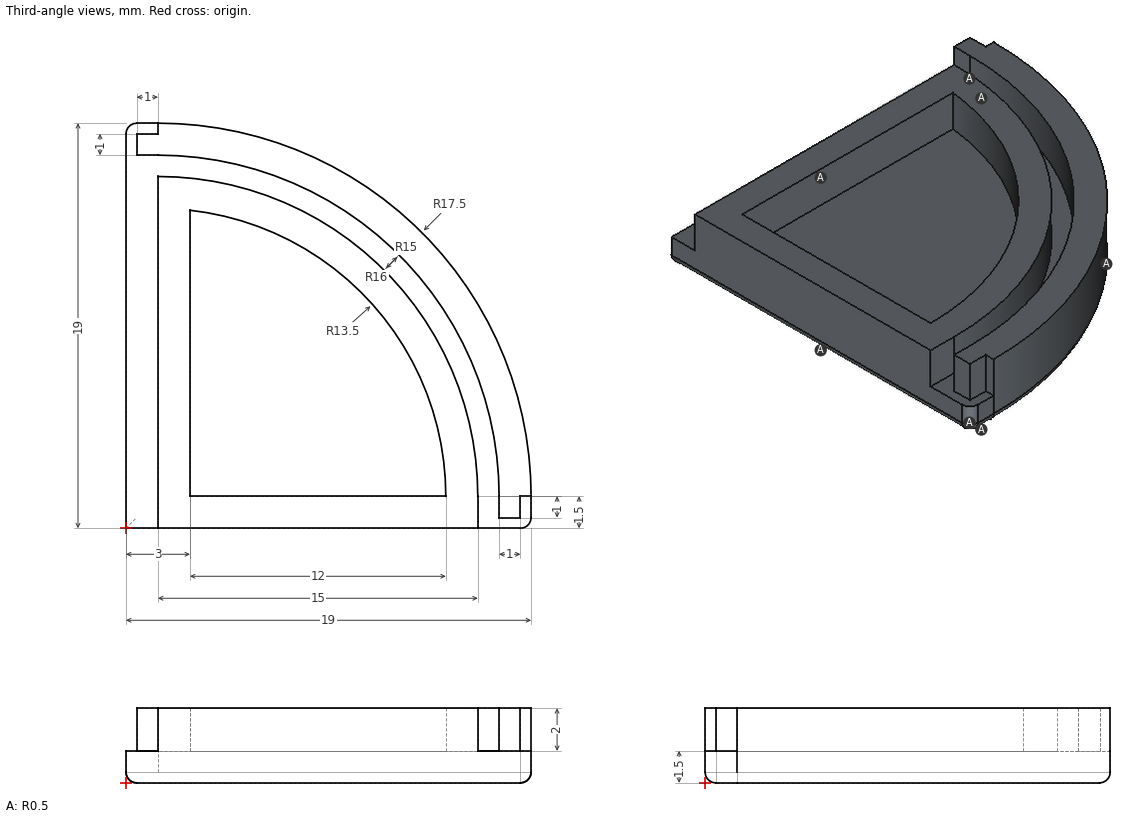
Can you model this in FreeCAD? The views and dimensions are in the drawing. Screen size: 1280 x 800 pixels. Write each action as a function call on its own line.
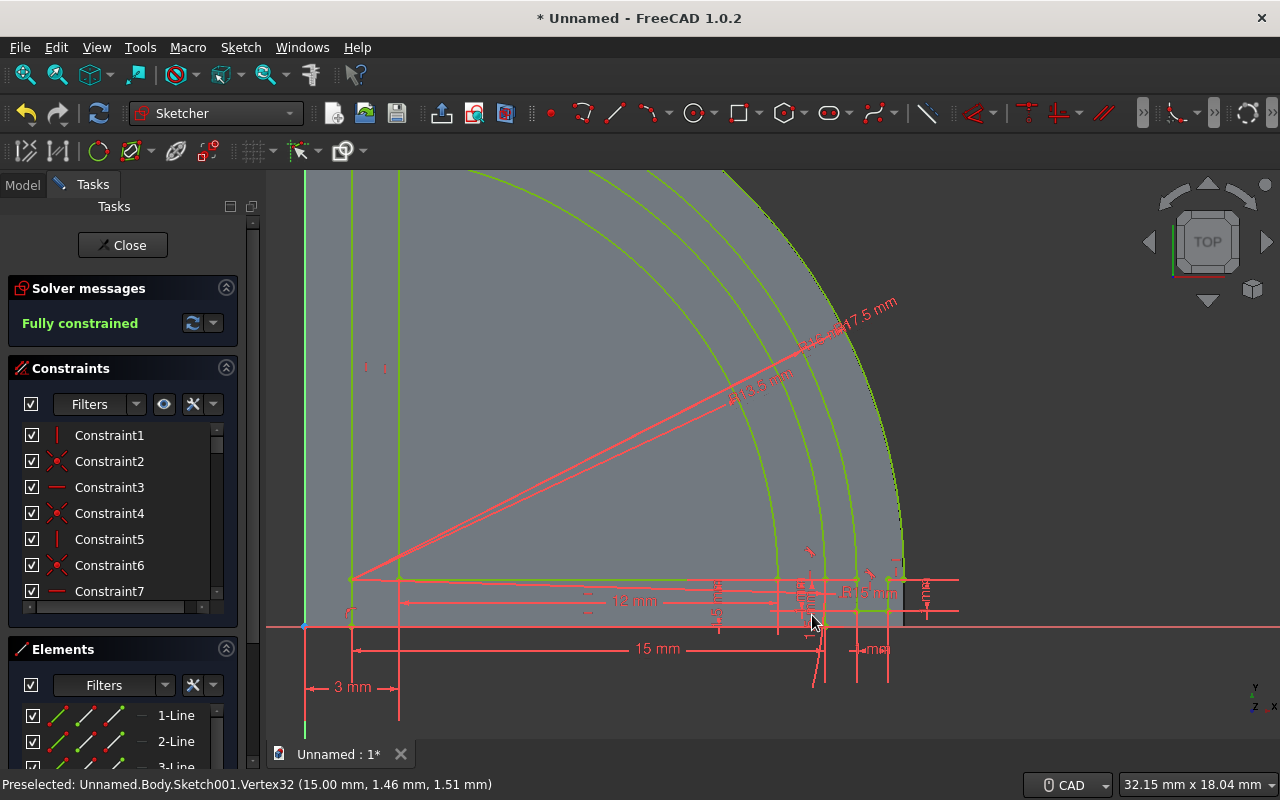
click(123, 245)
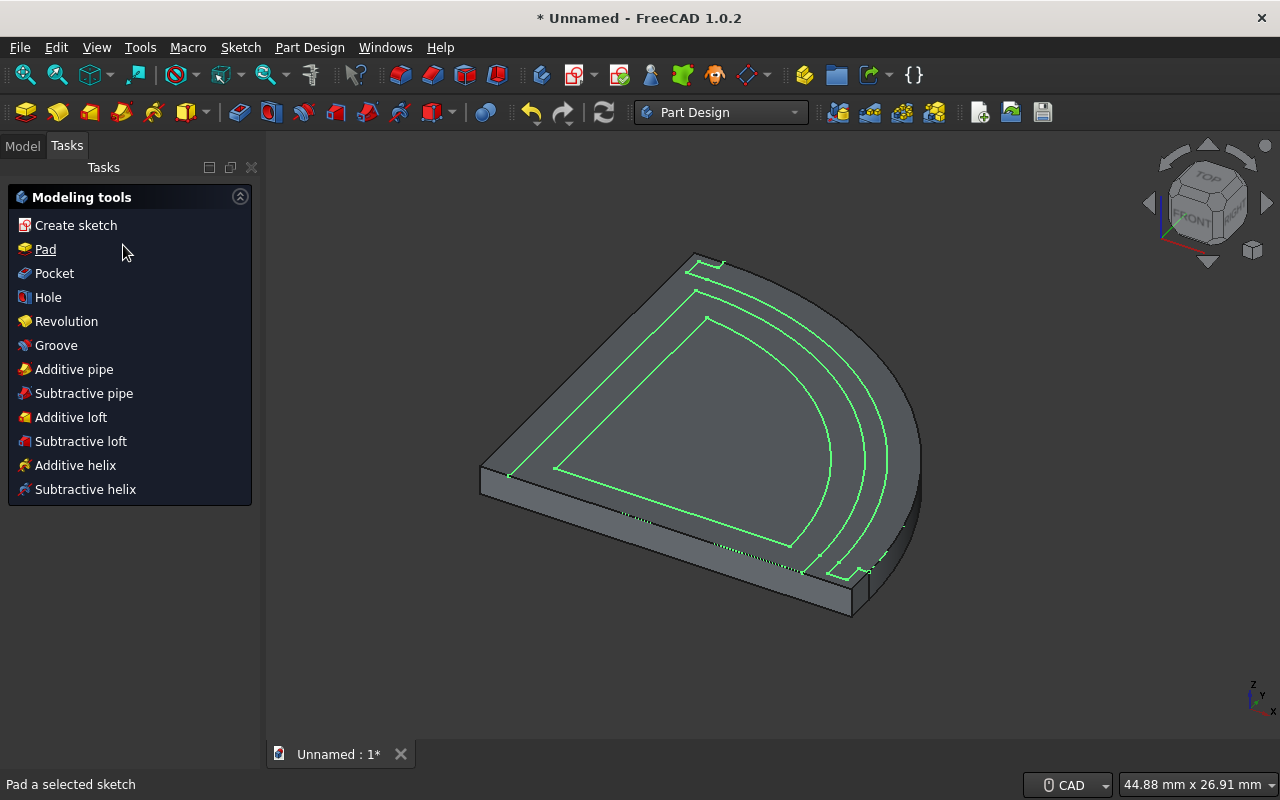
click(26, 112)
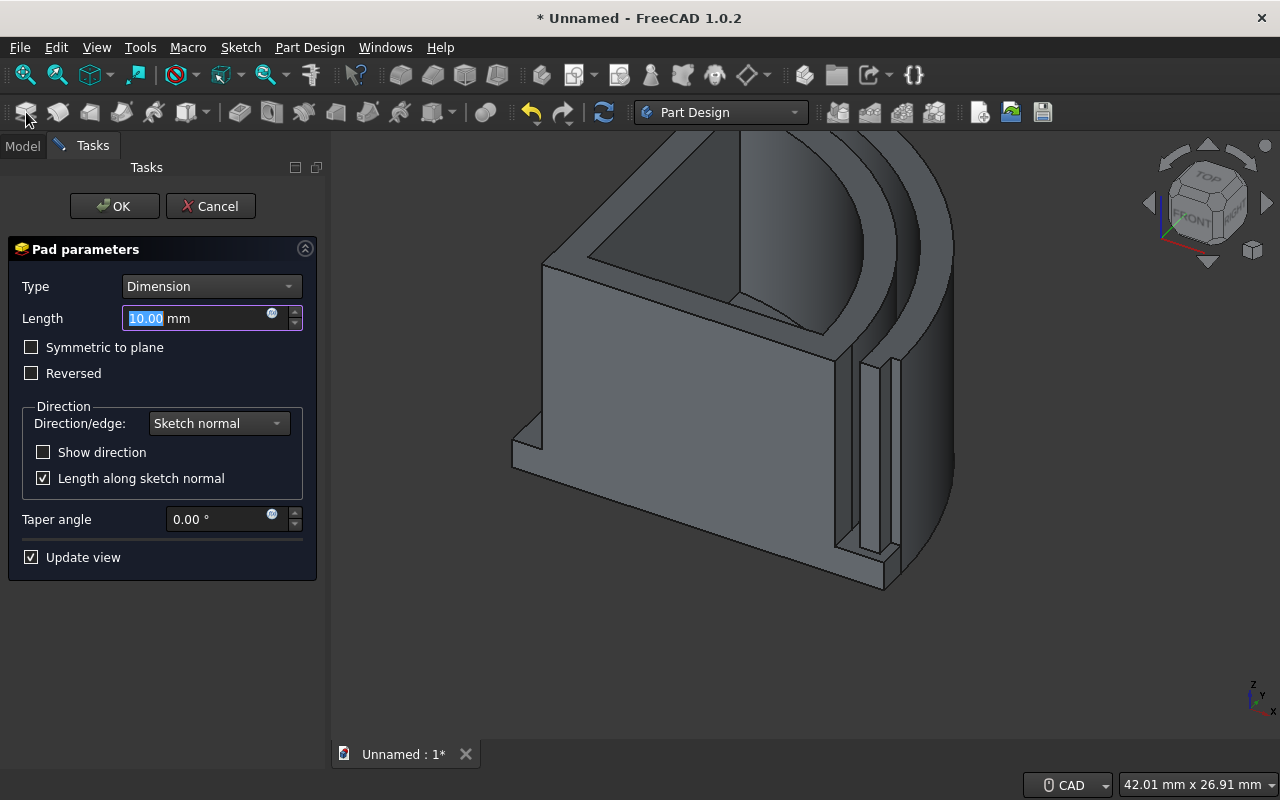
text(2)
key(Tab)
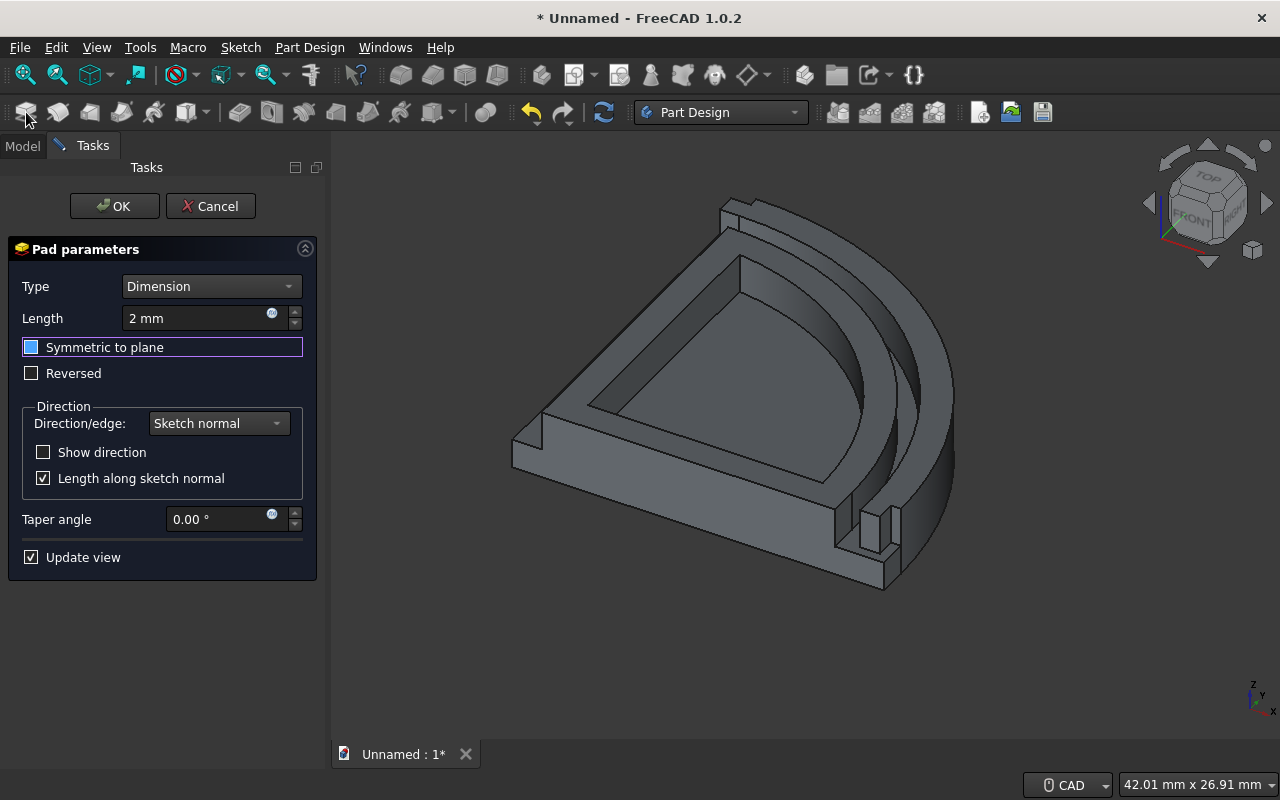
click(115, 206)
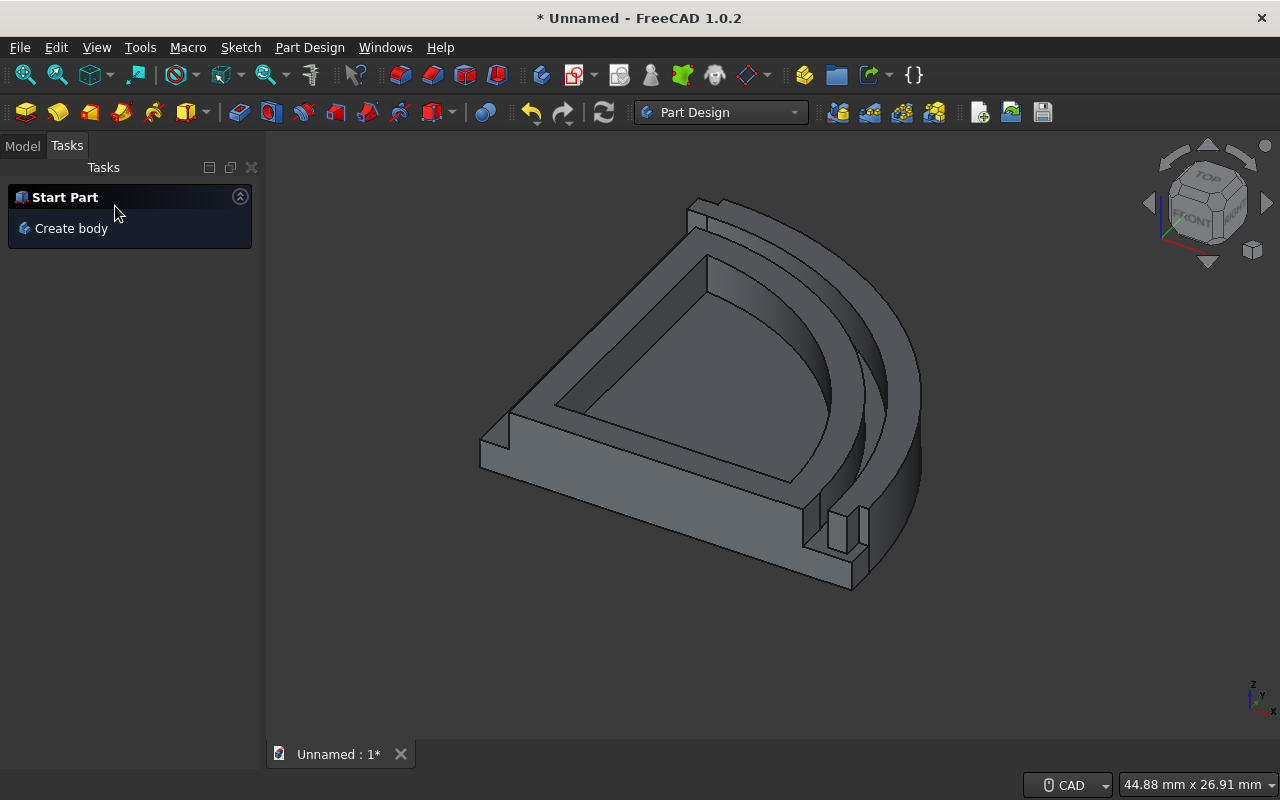
click(852, 576)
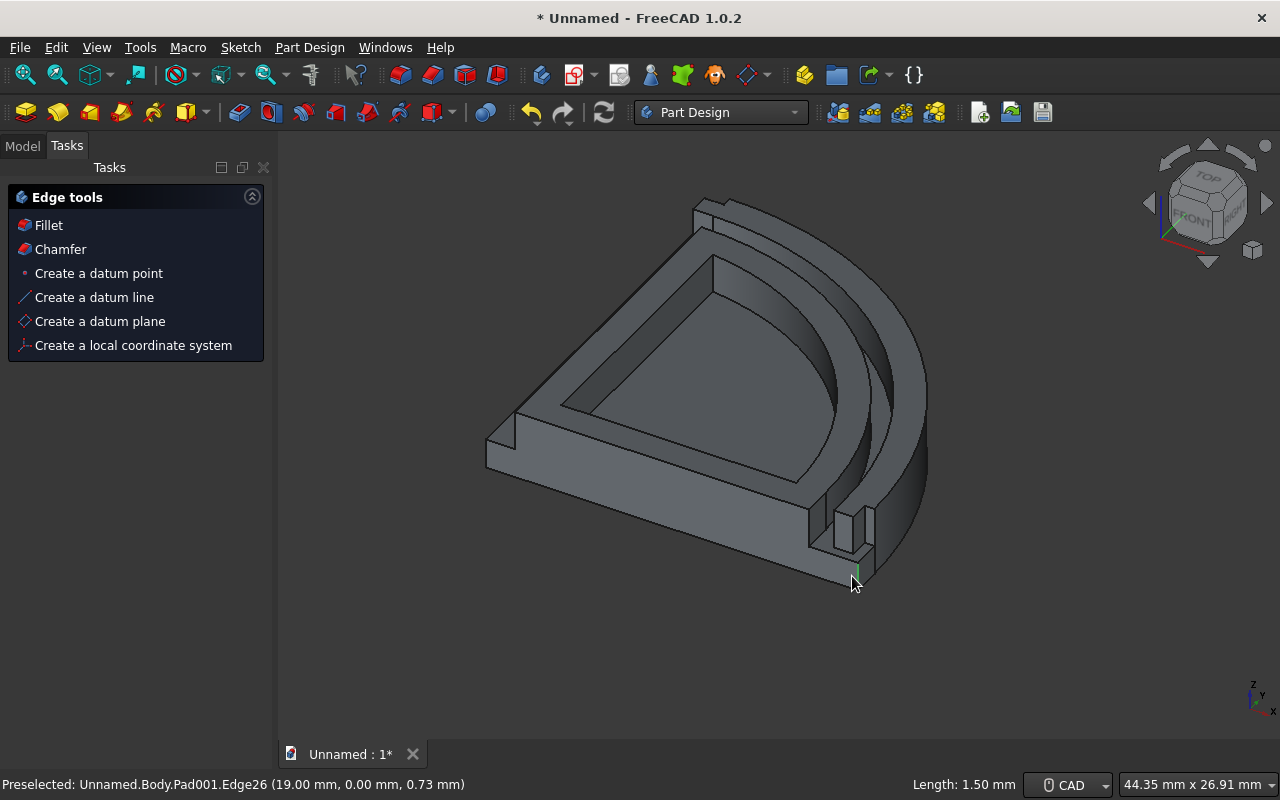
key(0)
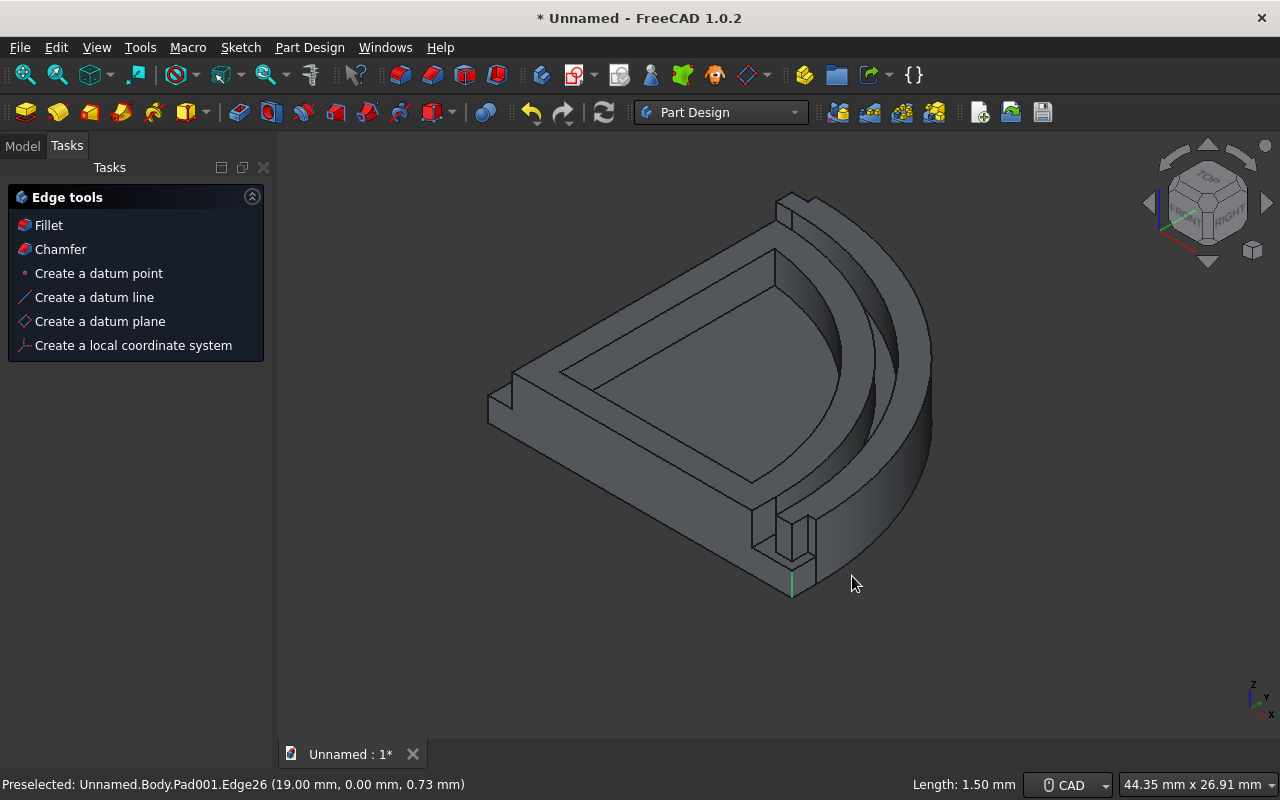
key(2)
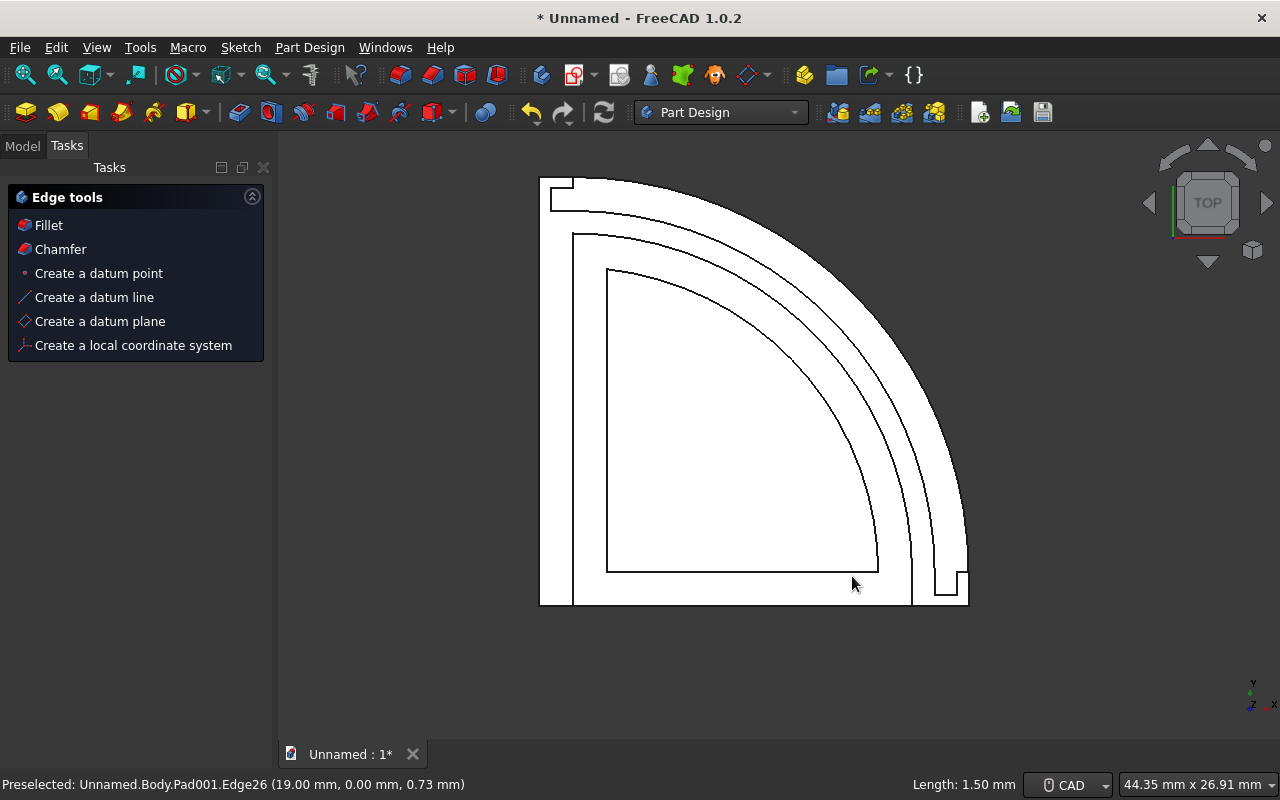
key(1)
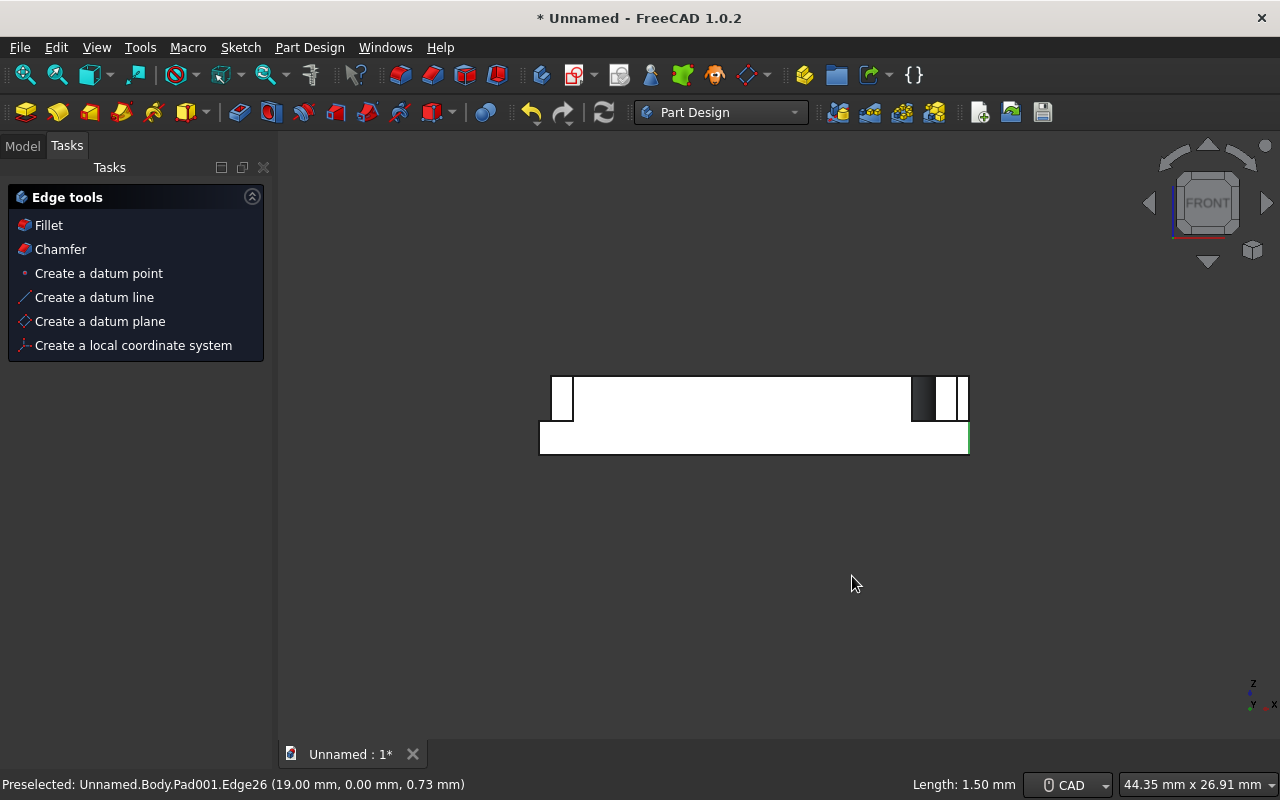
click(26, 76)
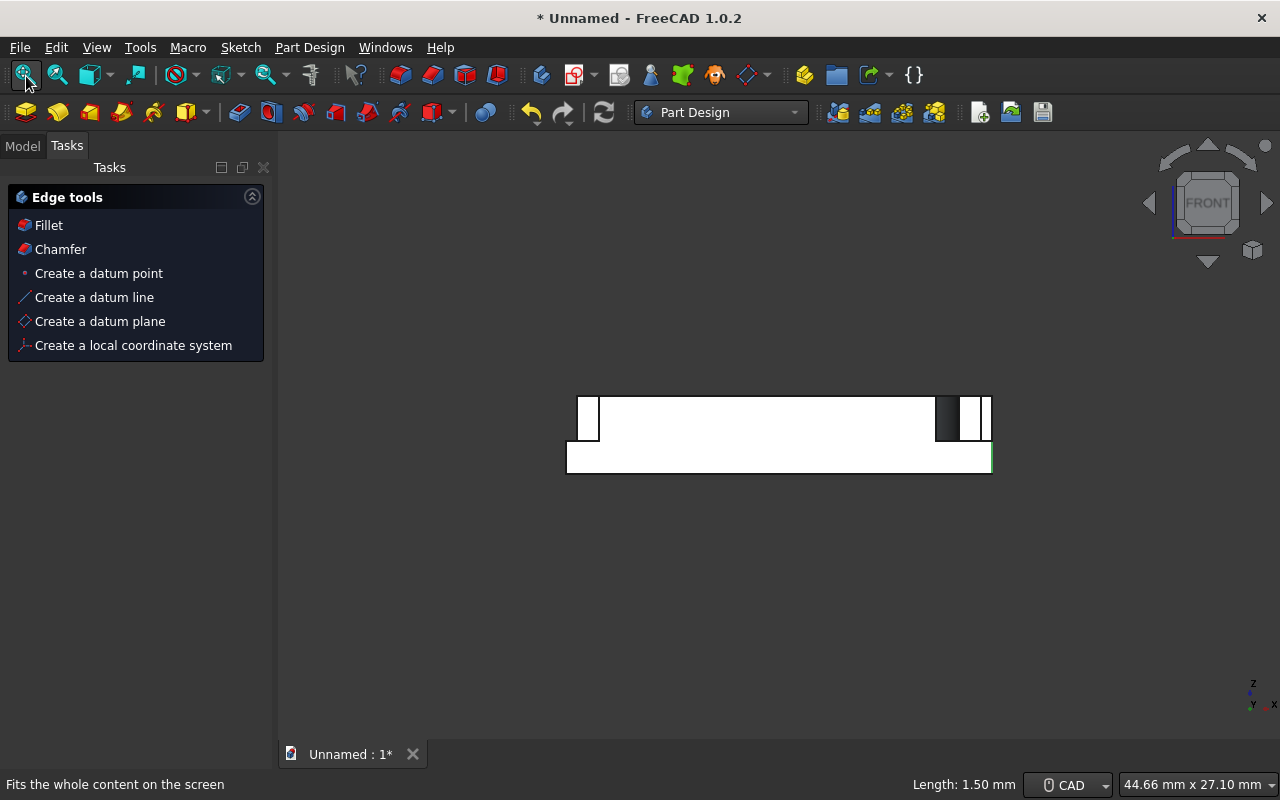
key(3)